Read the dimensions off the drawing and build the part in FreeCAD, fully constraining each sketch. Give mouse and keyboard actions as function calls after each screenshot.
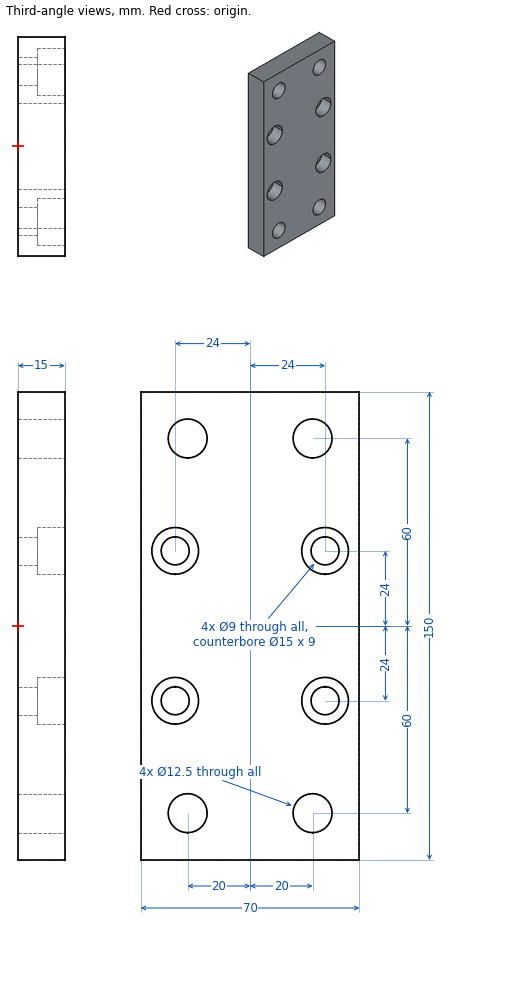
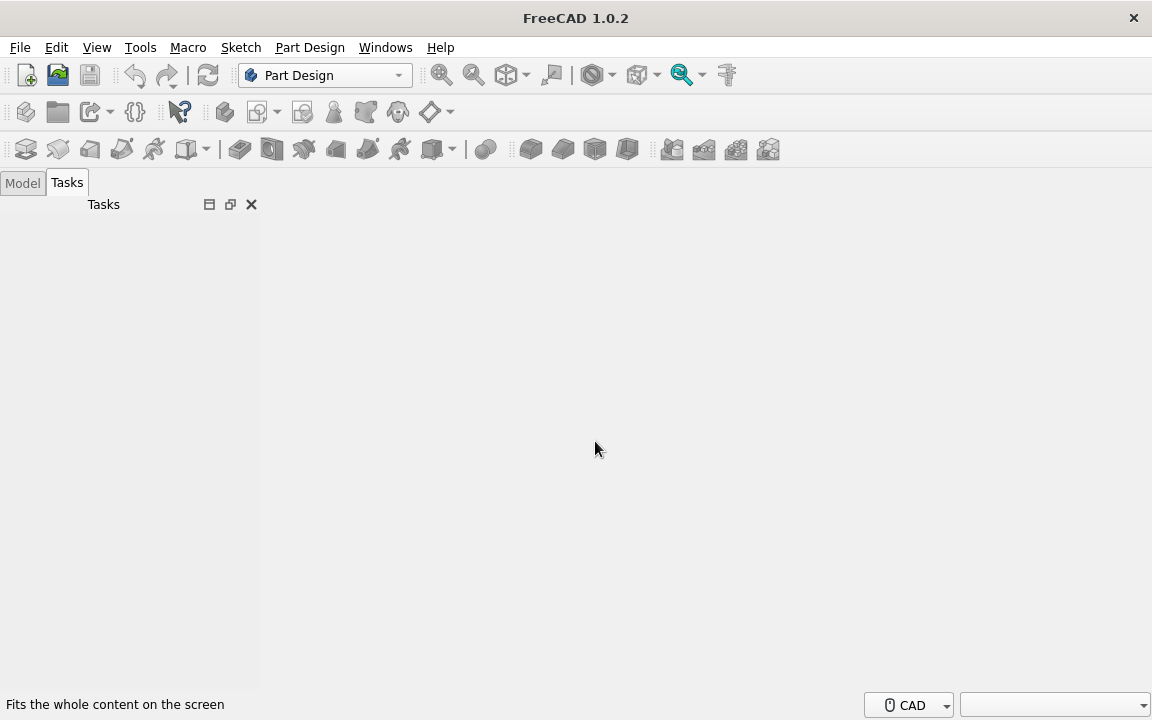
click(26, 76)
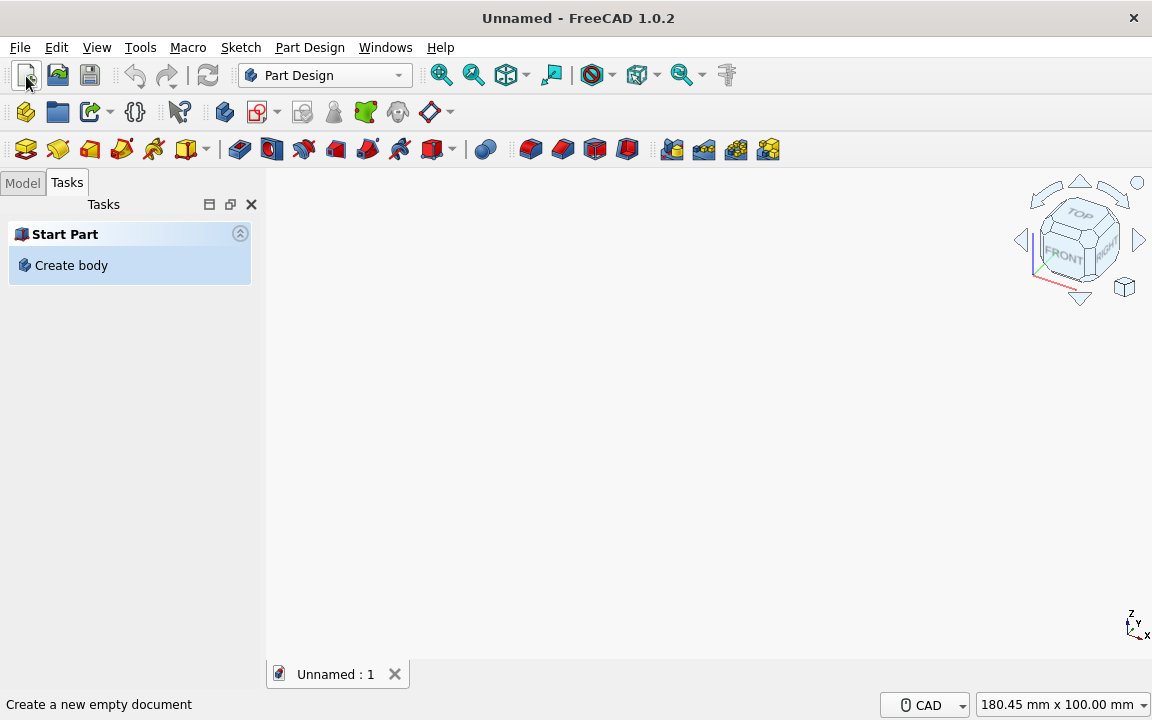
click(258, 112)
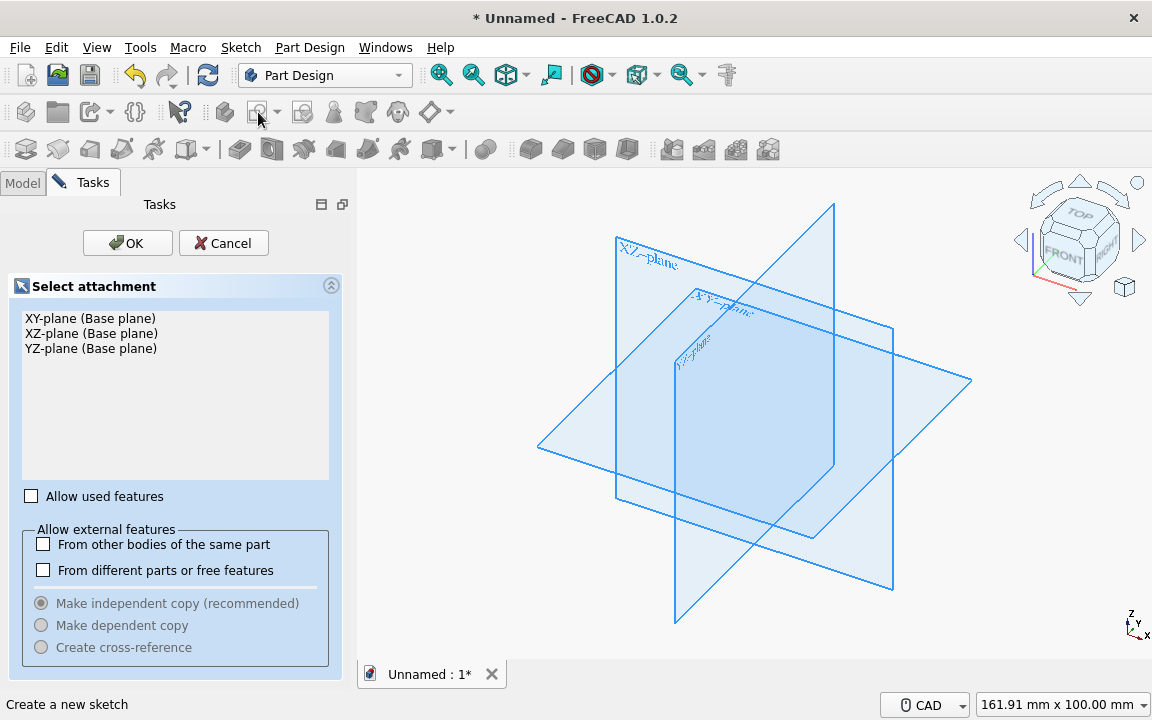
click(82, 348)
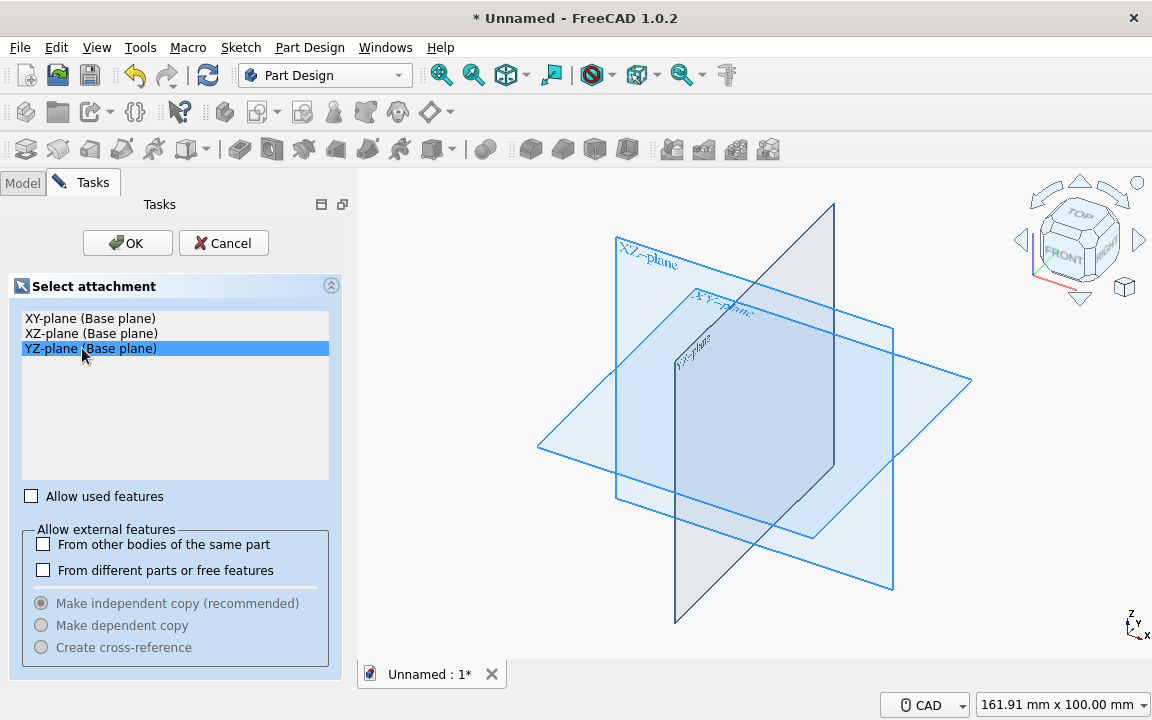
click(128, 243)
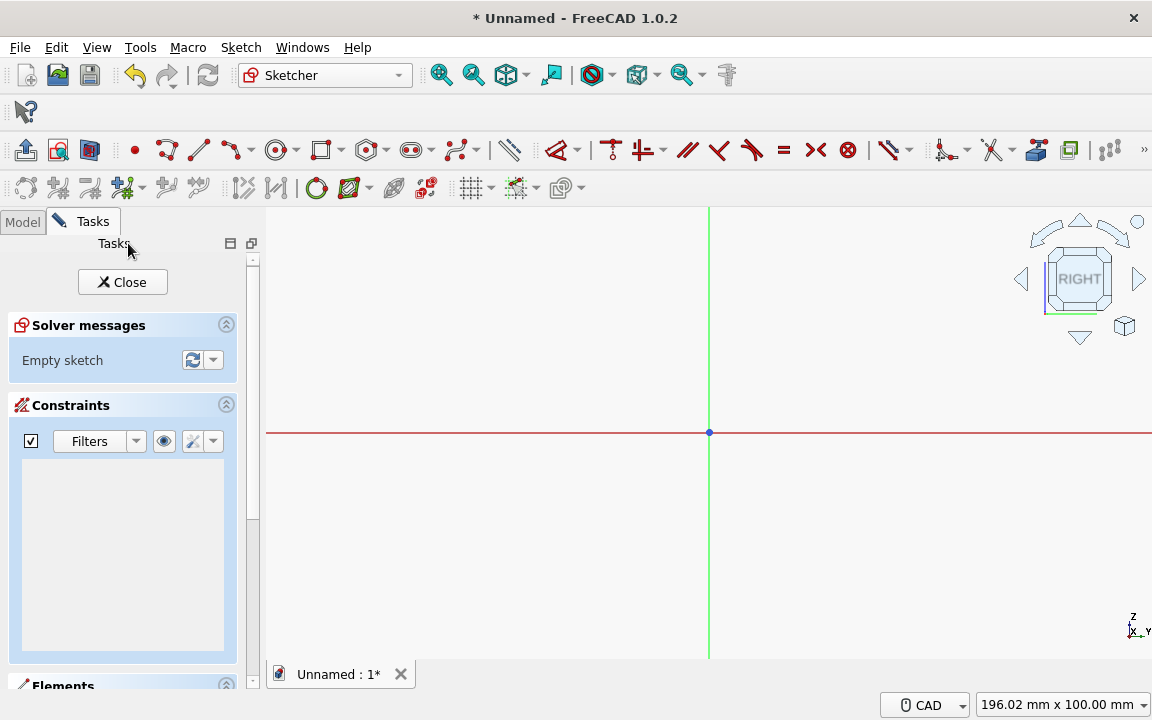
scroll(585, 433, down, 4)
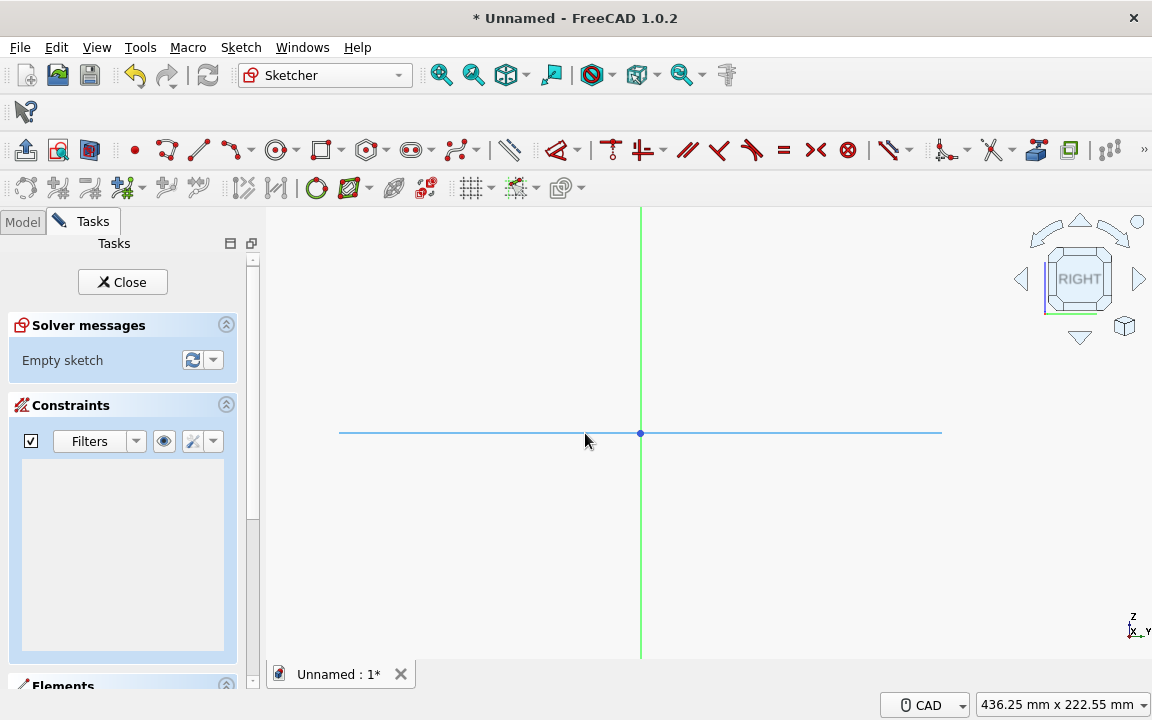
key(g)
key(v)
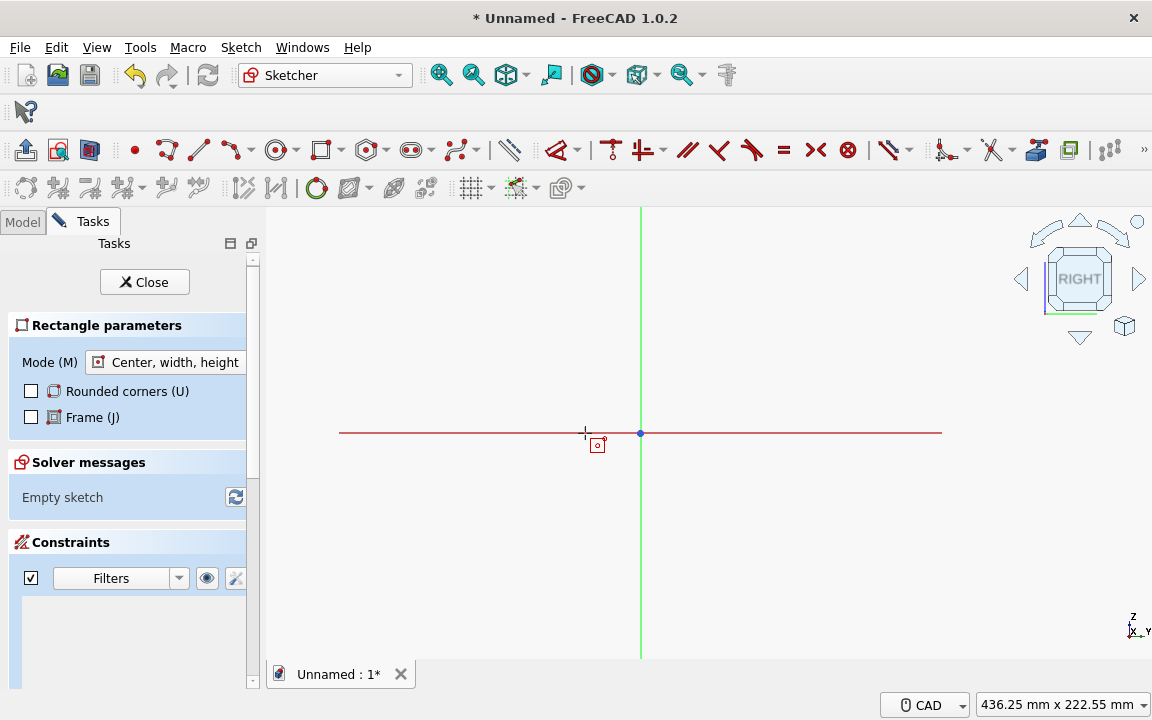
click(641, 433)
click(712, 281)
key(Escape)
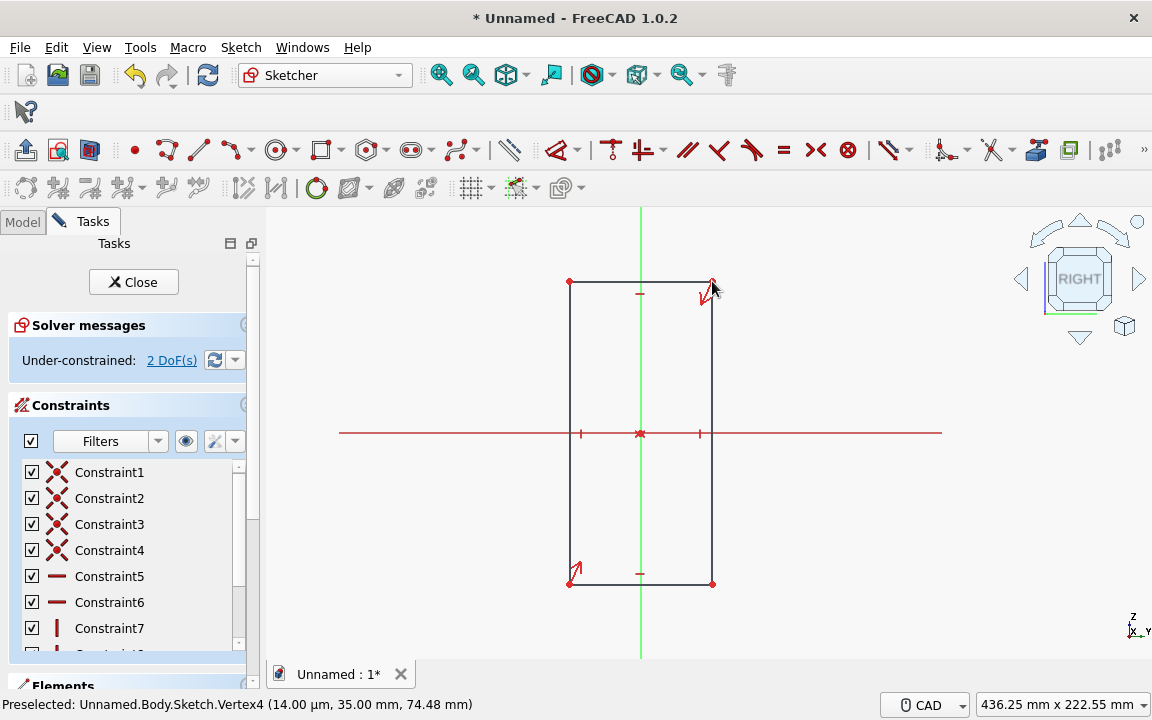
click(556, 150)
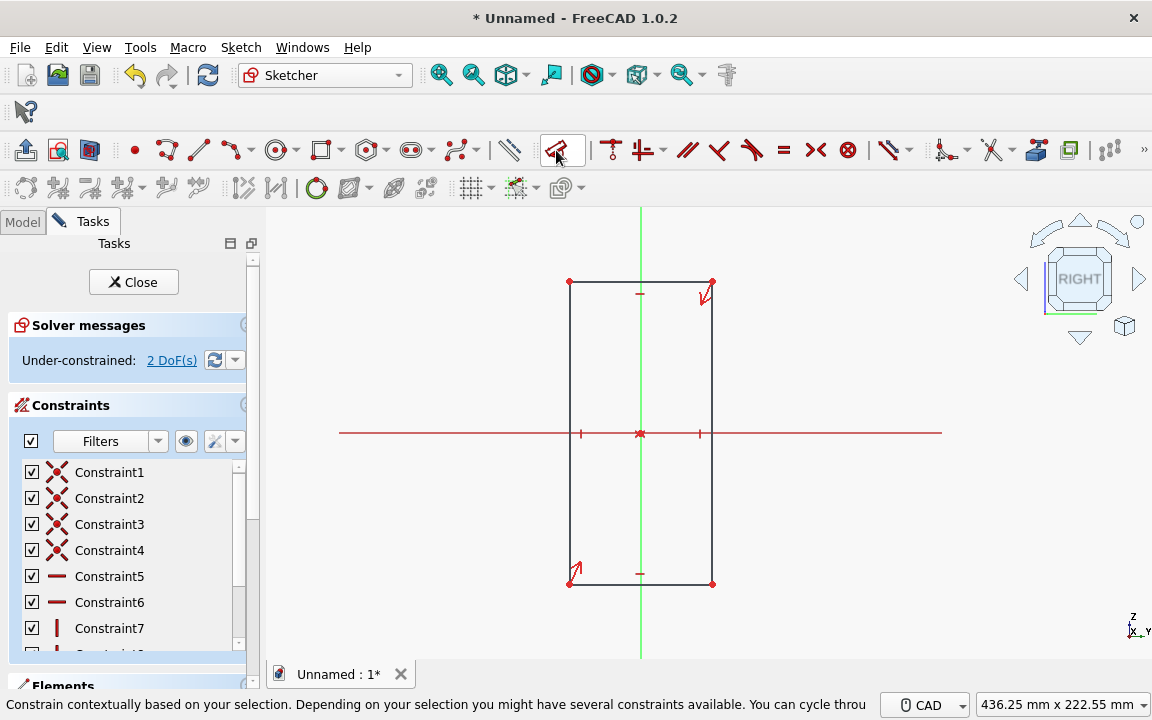
click(612, 585)
click(608, 619)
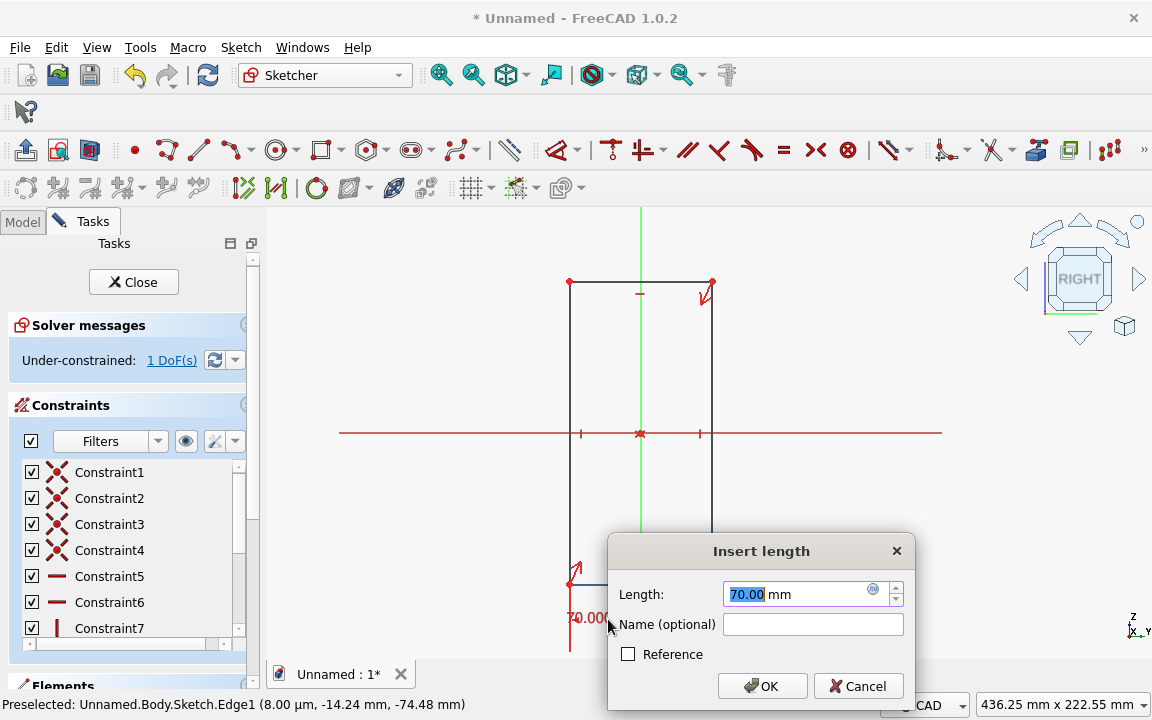
text(70)
key(Return)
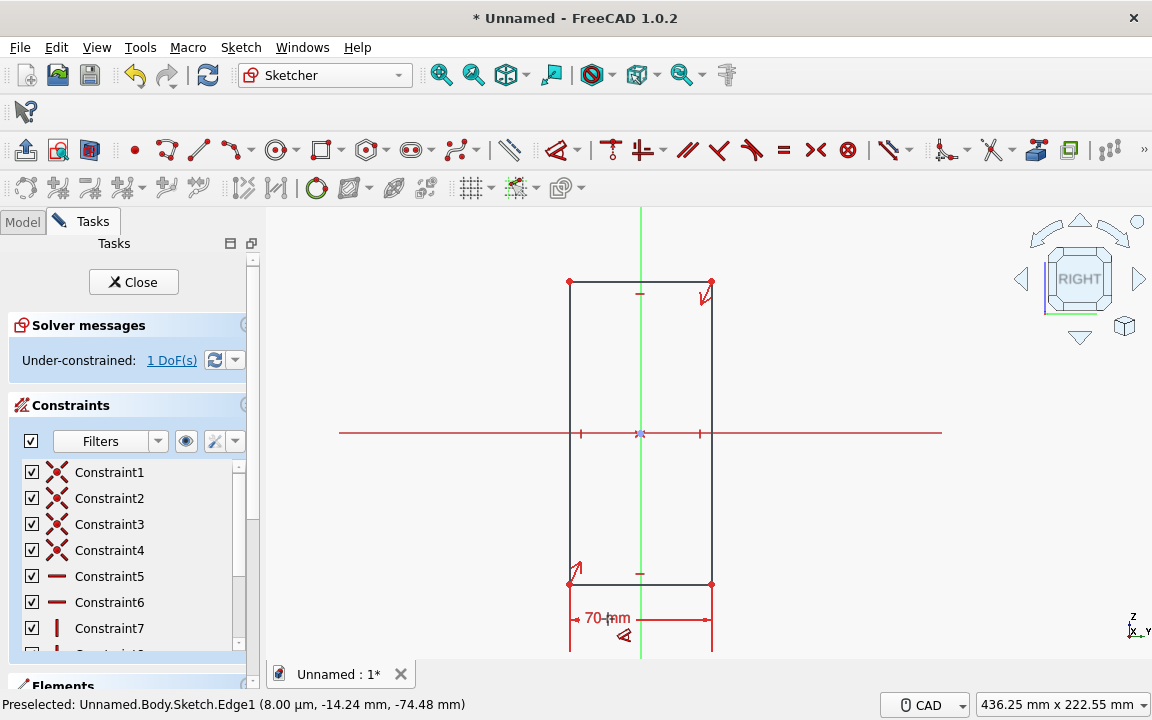
click(712, 494)
click(746, 364)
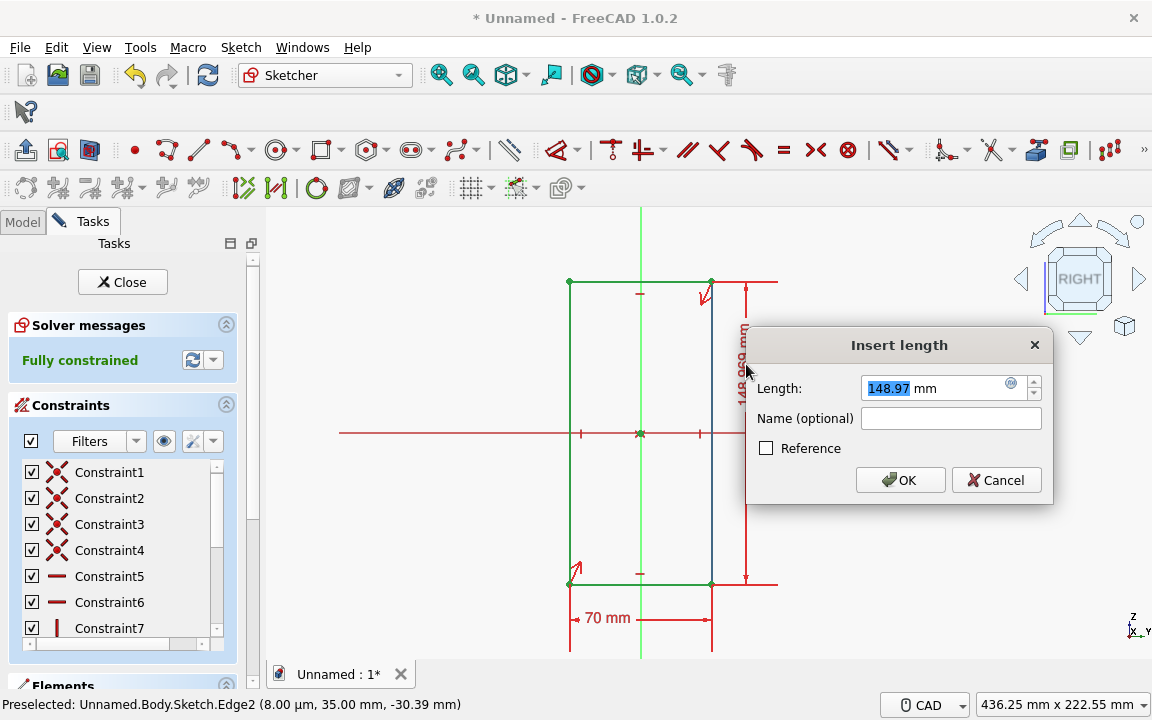
text(150)
key(Return)
key(Escape)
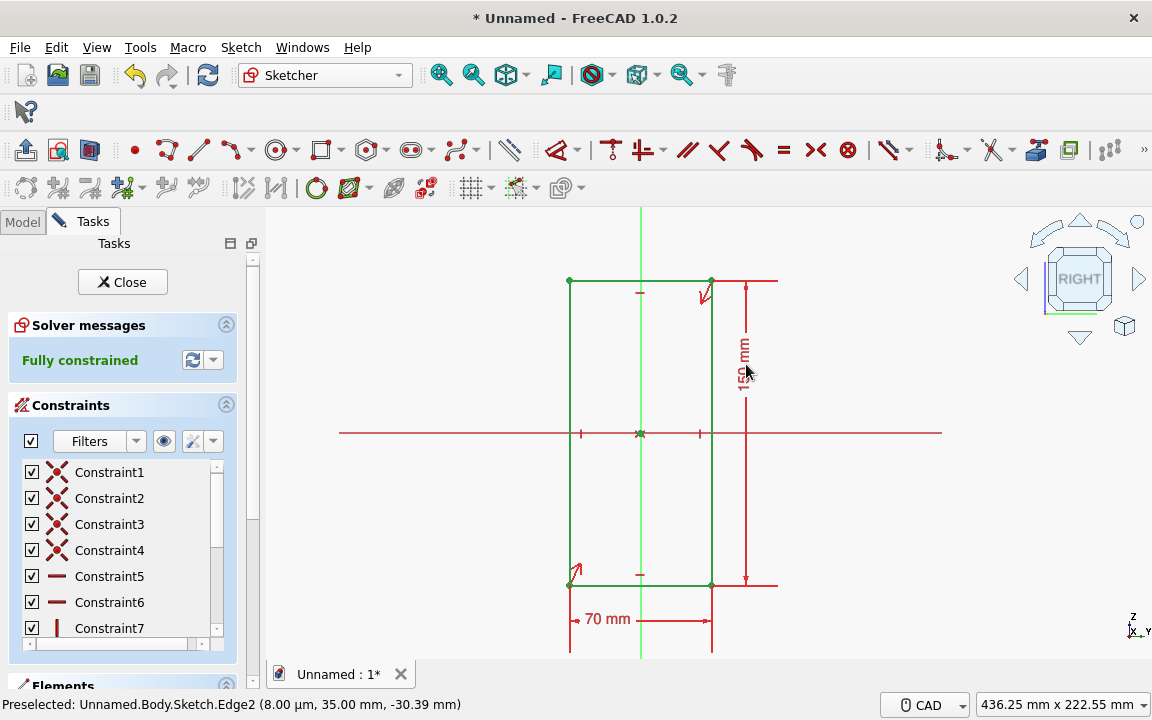
click(123, 282)